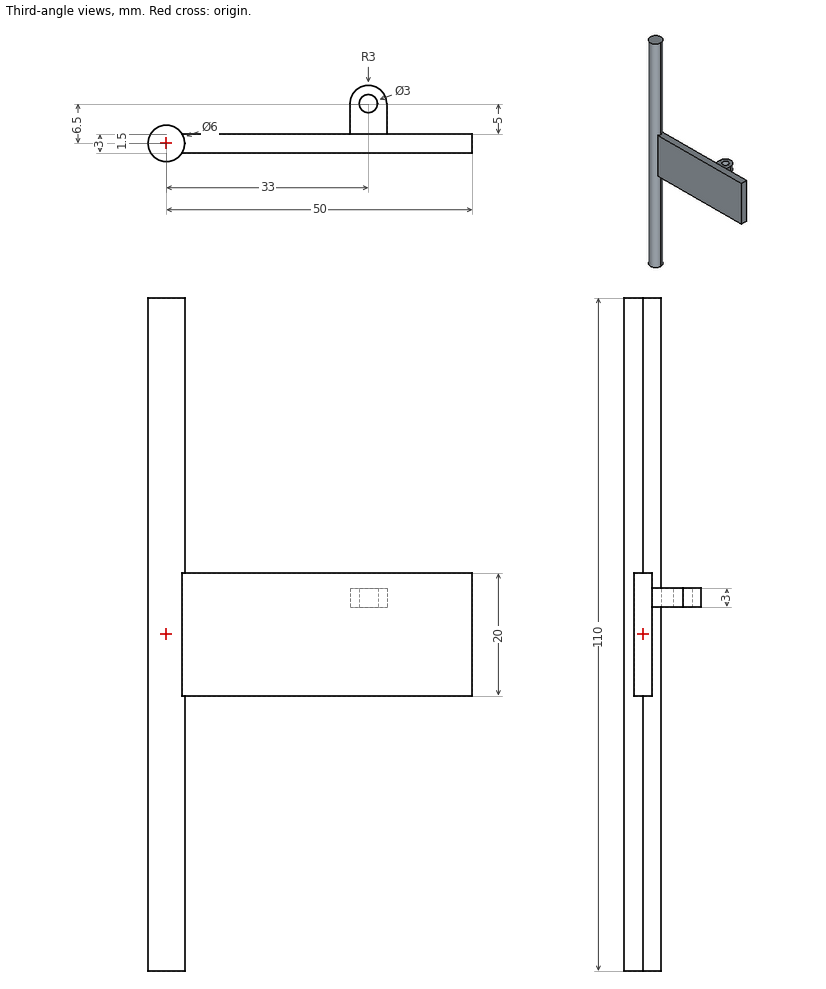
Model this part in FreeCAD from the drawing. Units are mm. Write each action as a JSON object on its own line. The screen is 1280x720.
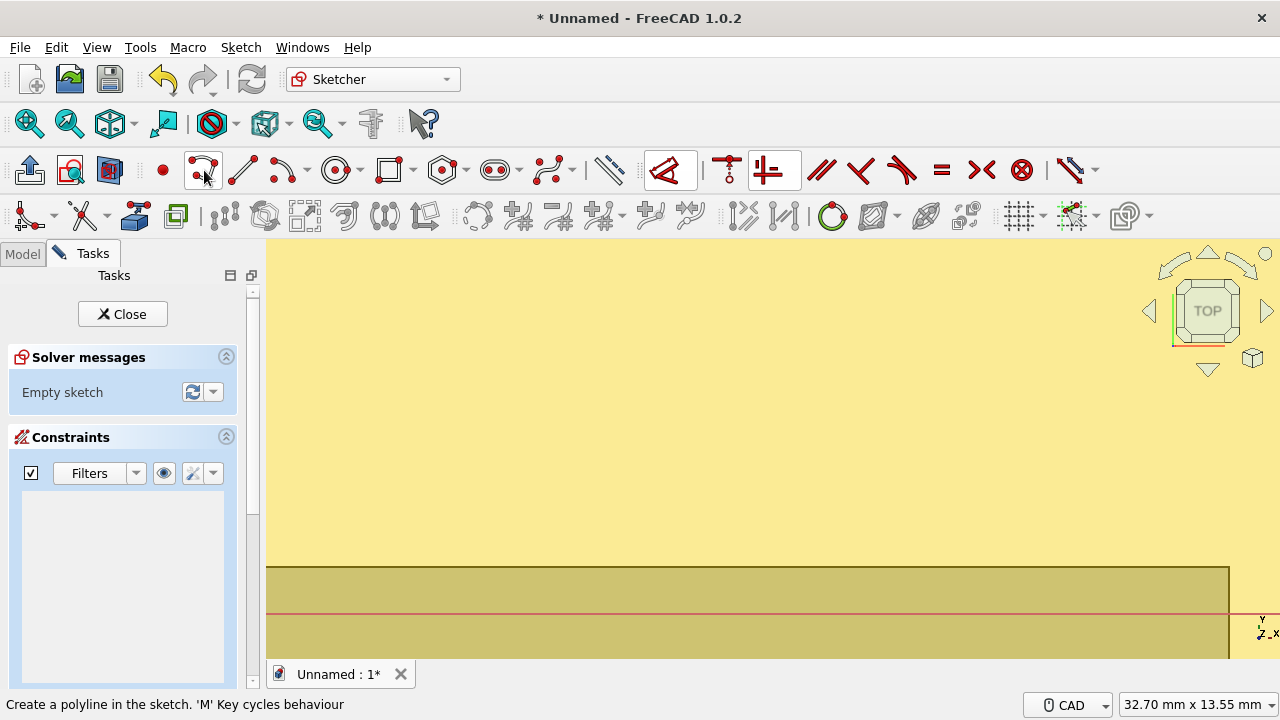
{"action": "left_click", "coordinate": [609, 412]}
{"action": "left_click", "coordinate": [609, 567]}
{"action": "left_click", "coordinate": [795, 567]}
{"action": "left_click", "coordinate": [795, 412]}
{"action": "right_click", "coordinate": [795, 412]}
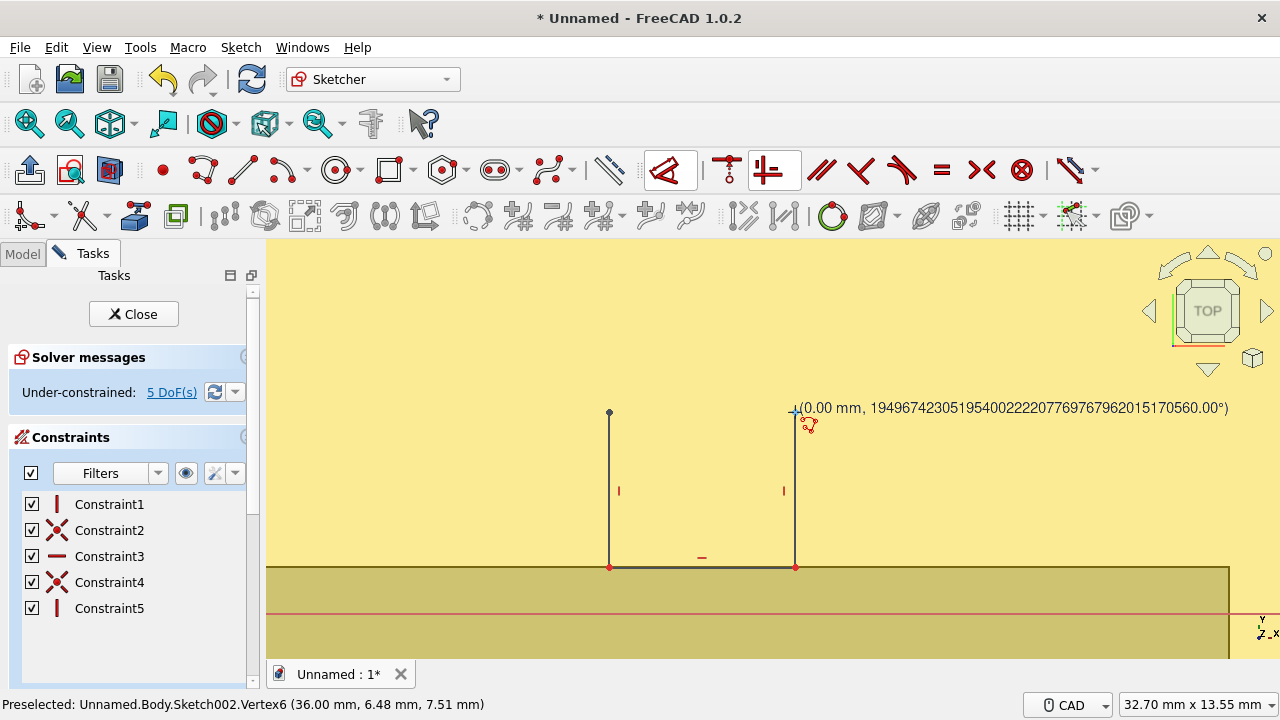
{"action": "key", "text": "g 3 a"}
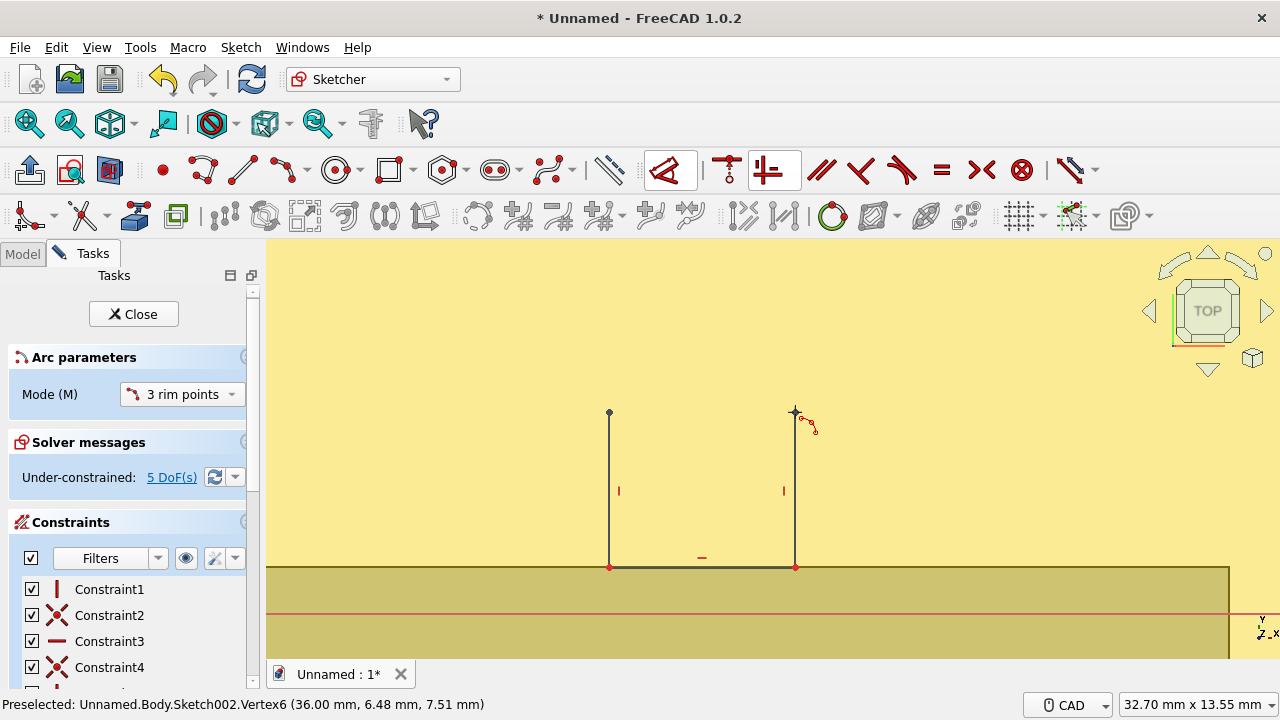
{"action": "left_click", "coordinate": [795, 413]}
{"action": "left_click", "coordinate": [609, 413]}
{"action": "left_click", "coordinate": [702, 319]}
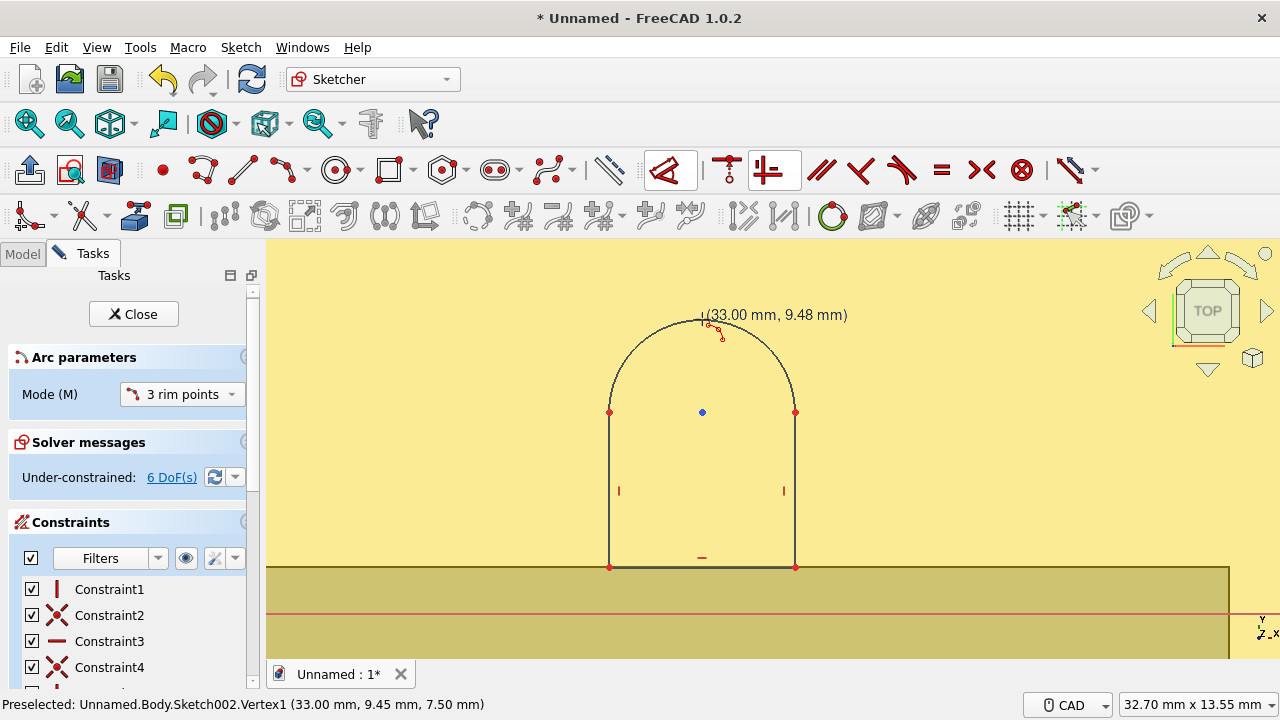
{"action": "left_click", "coordinate": [336, 170]}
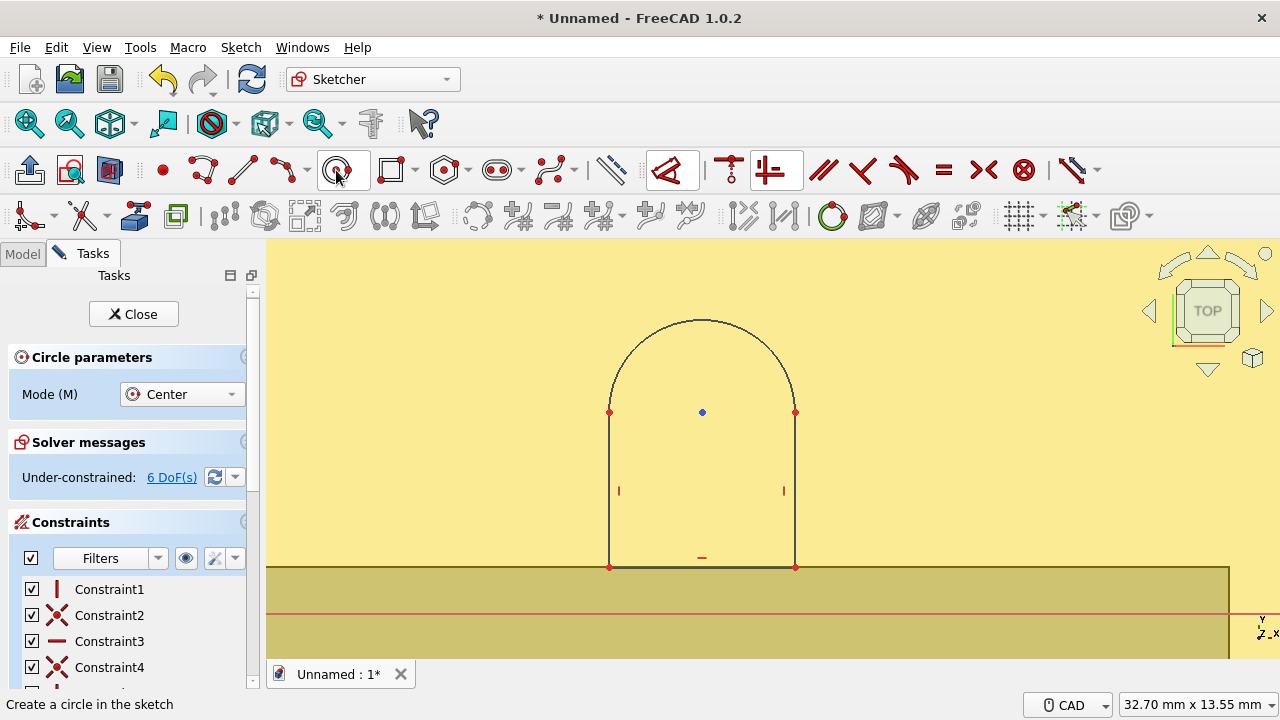
{"action": "left_click", "coordinate": [702, 412]}
{"action": "left_click", "coordinate": [735, 379]}
{"action": "key", "text": "Escape"}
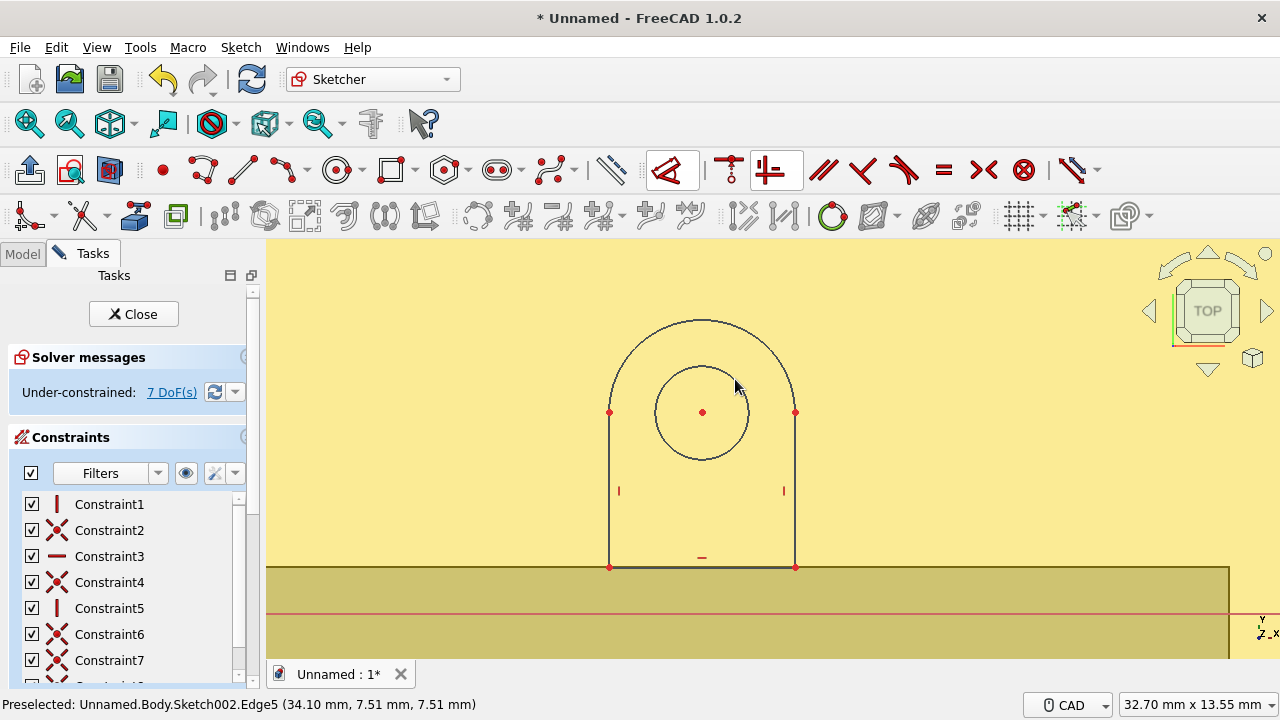
{"action": "left_click", "coordinate": [609, 460]}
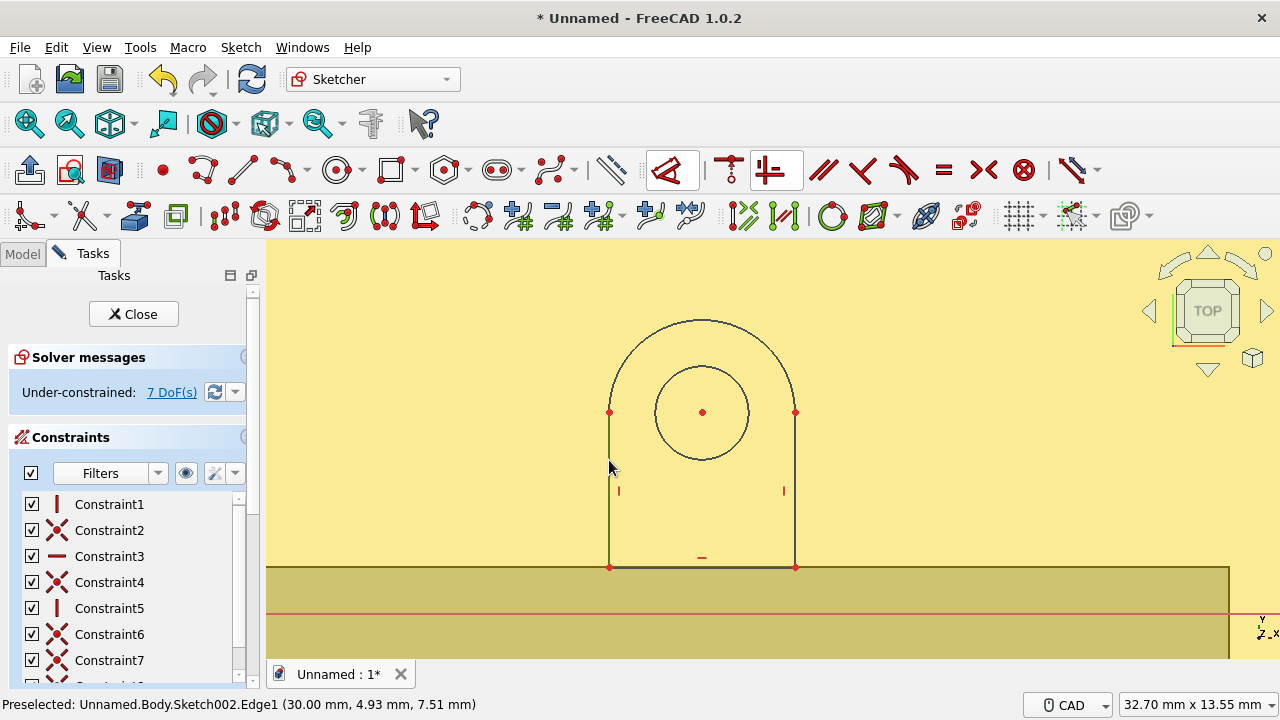
{"action": "left_click", "coordinate": [757, 338]}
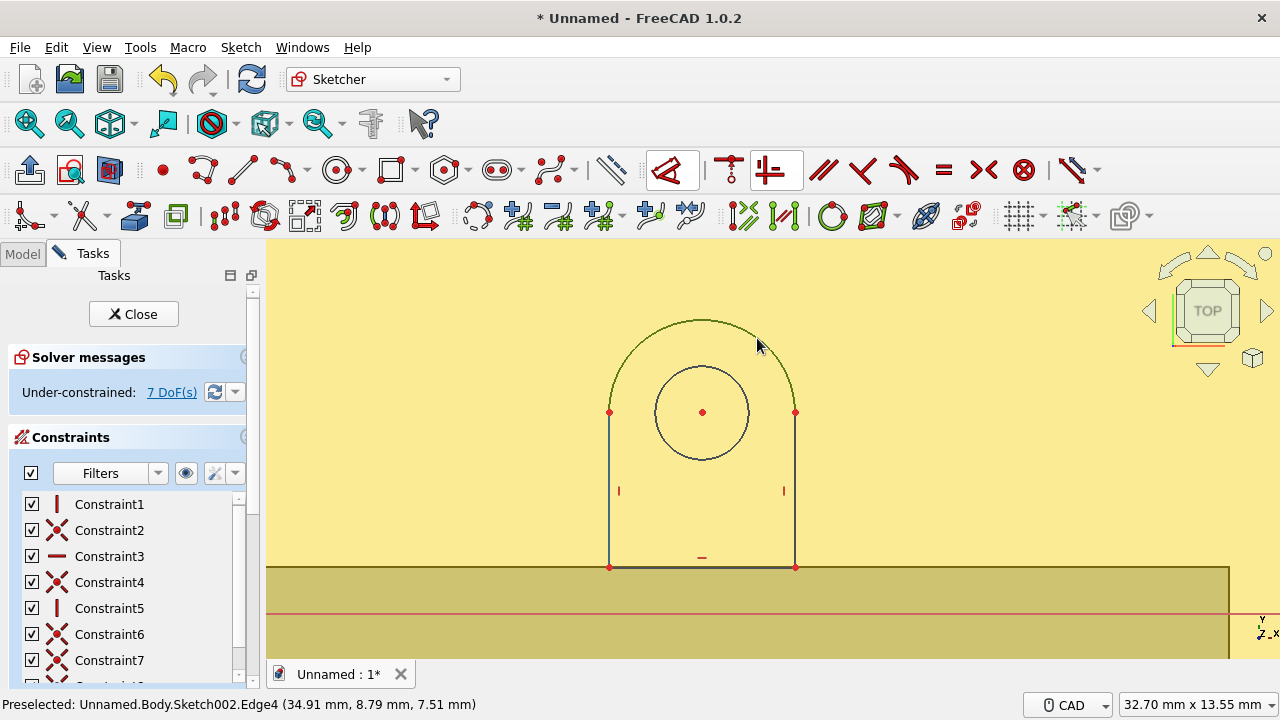
{"action": "left_click", "coordinate": [904, 170]}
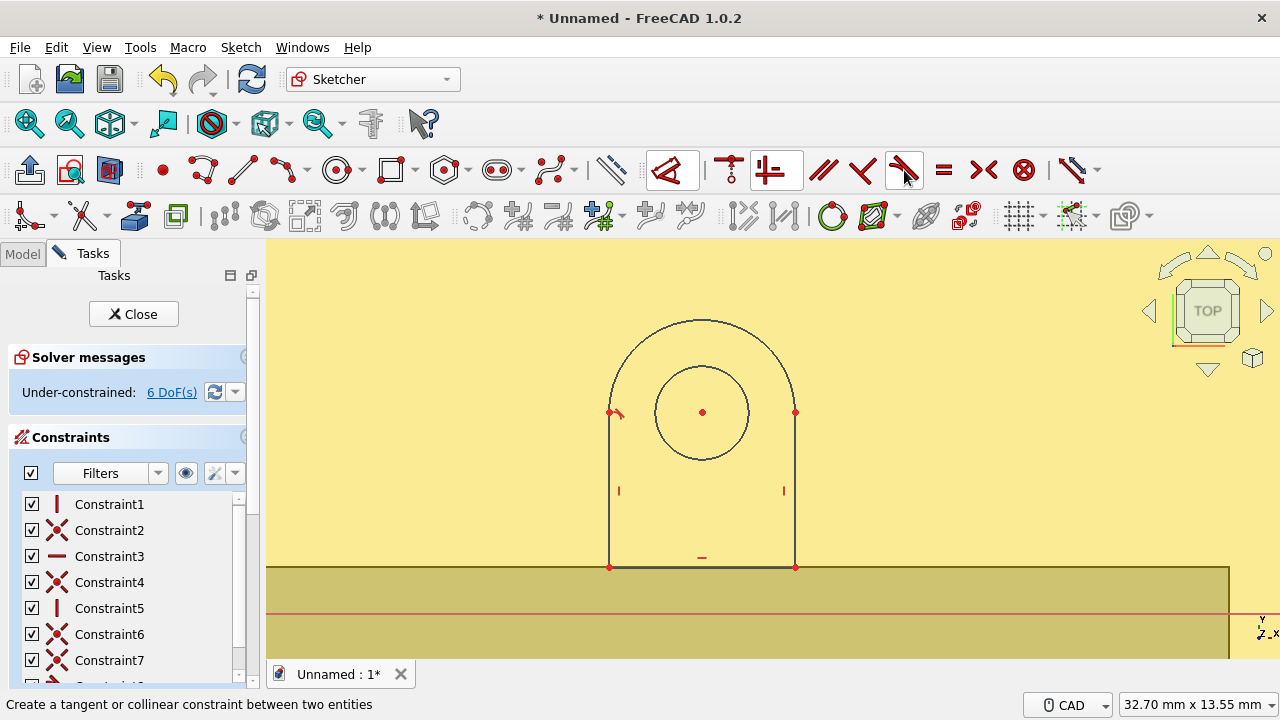
{"action": "left_click", "coordinate": [795, 521]}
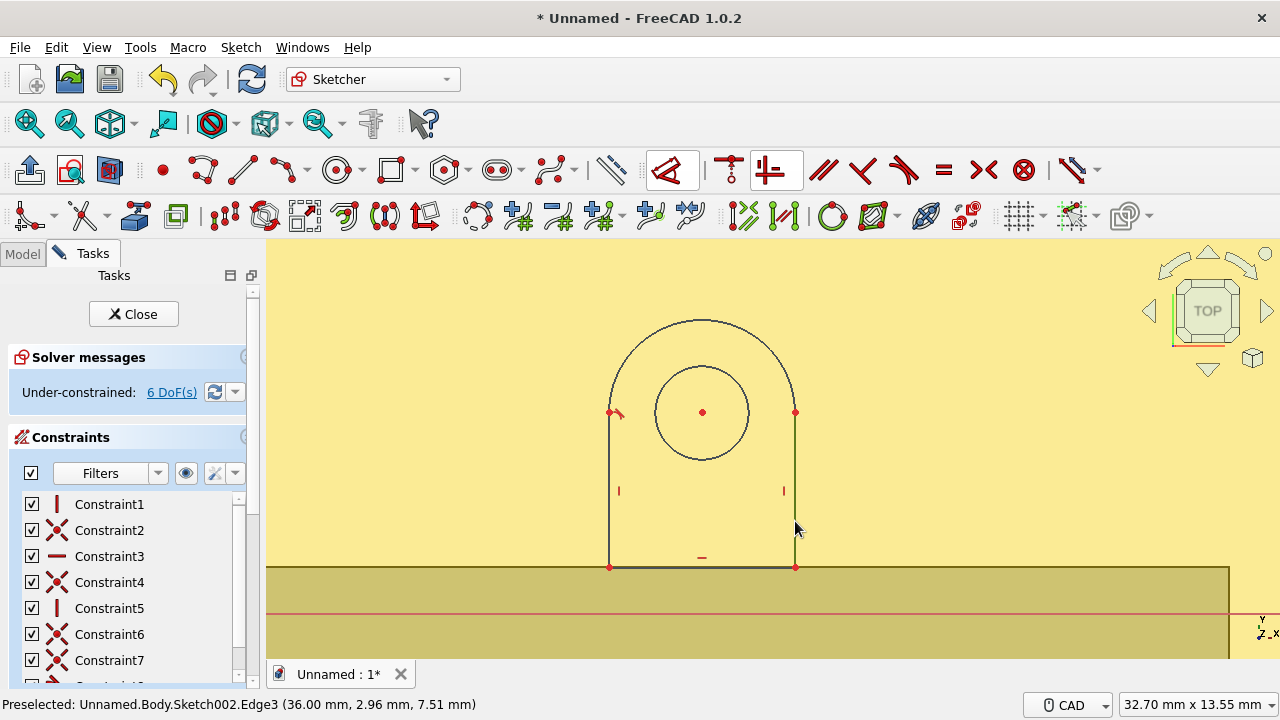
{"action": "left_click", "coordinate": [757, 338]}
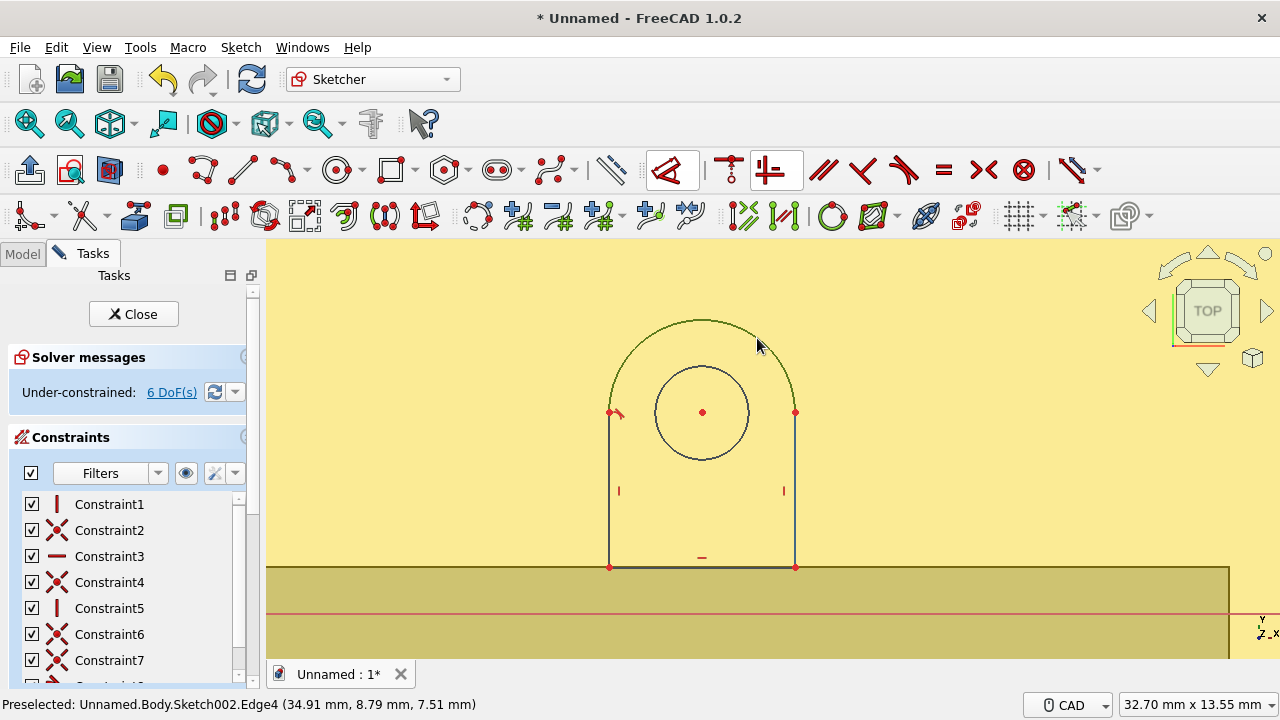
{"action": "left_click", "coordinate": [904, 170]}